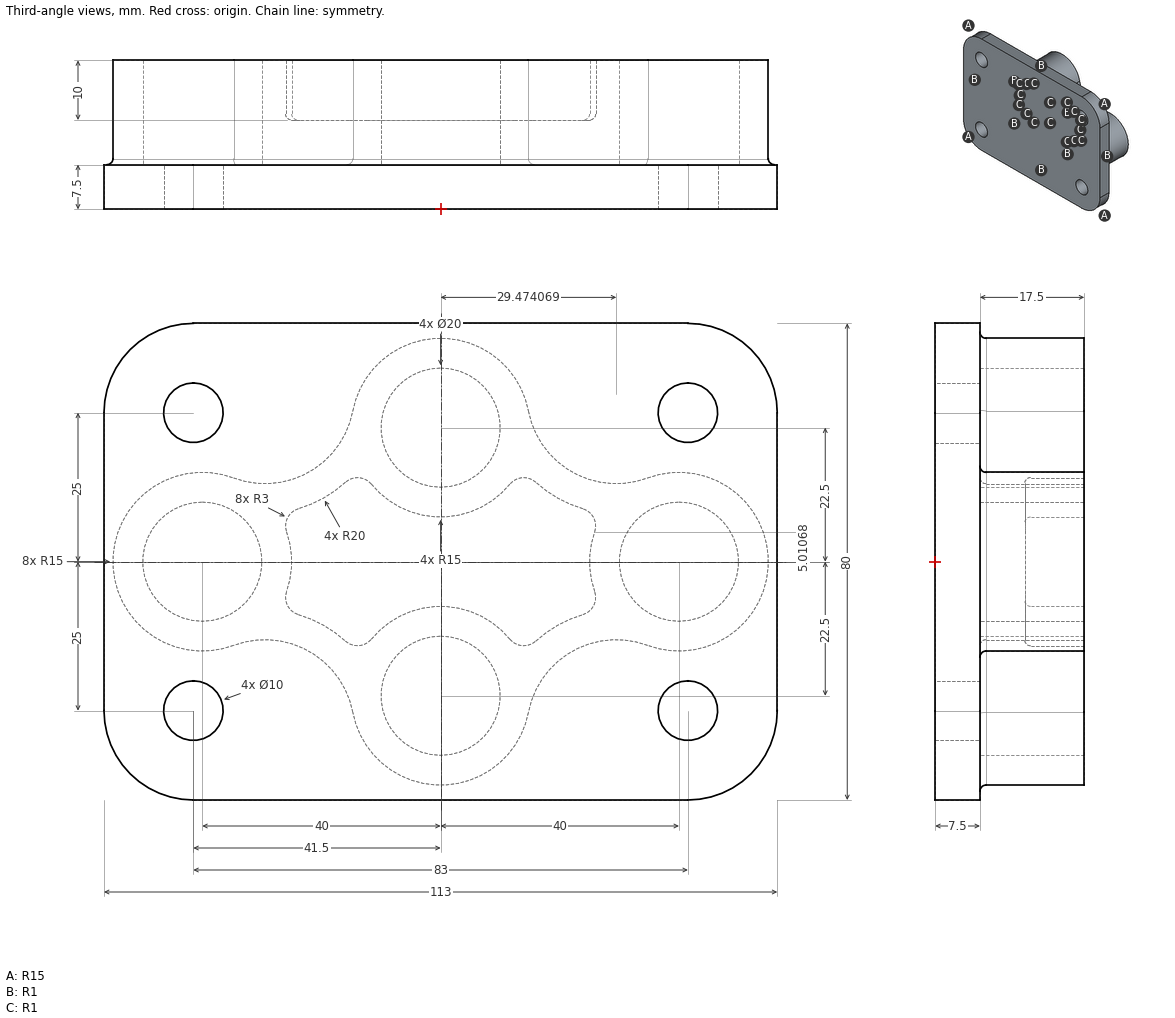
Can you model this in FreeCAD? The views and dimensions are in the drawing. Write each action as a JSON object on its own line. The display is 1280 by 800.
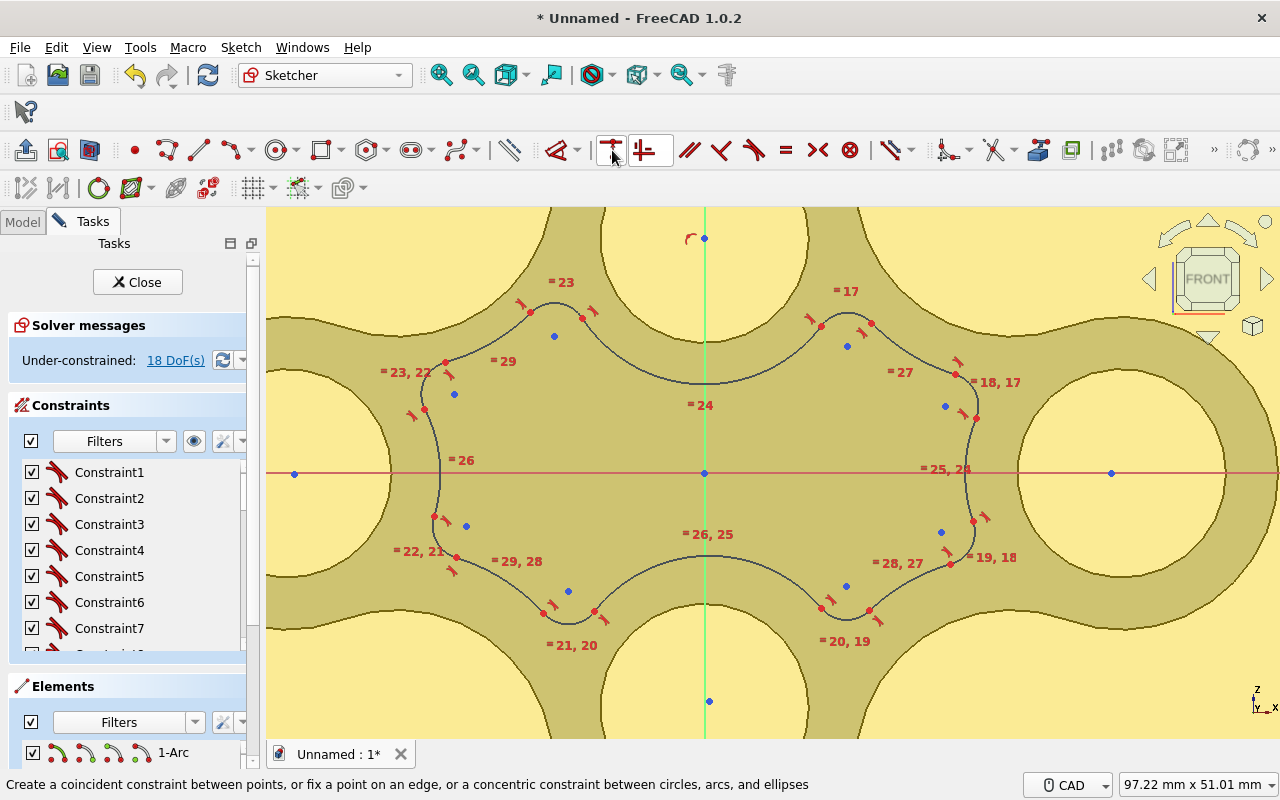
{"action": "left_click", "coordinate": [1111, 474]}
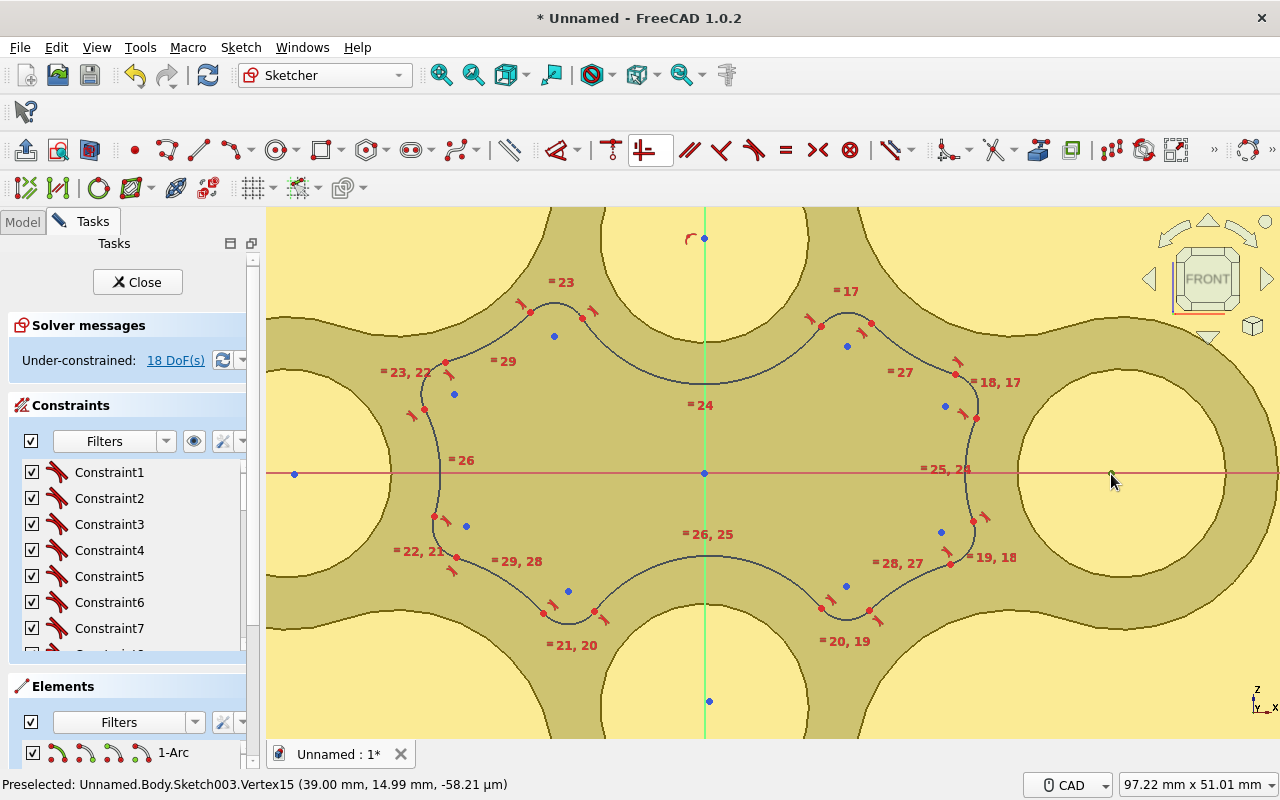
{"action": "left_click", "coordinate": [353, 473]}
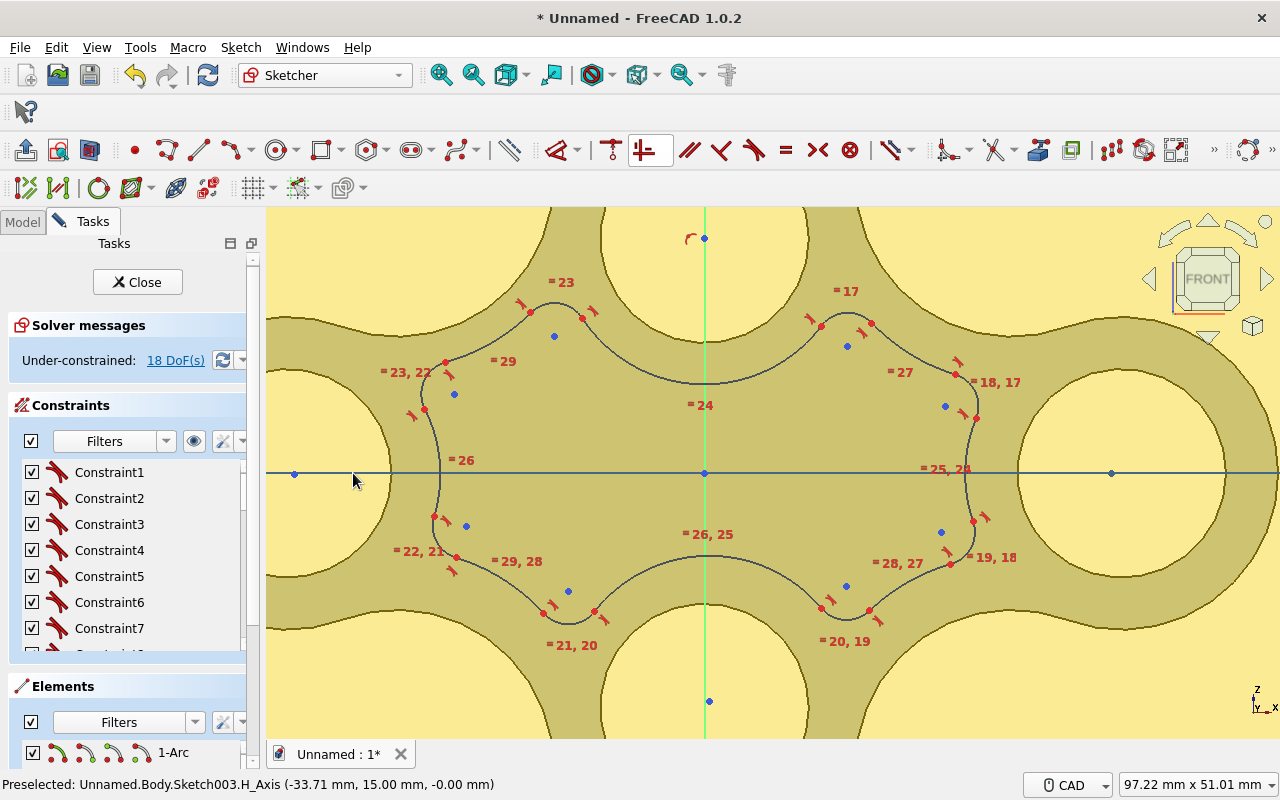
{"action": "key", "text": "c"}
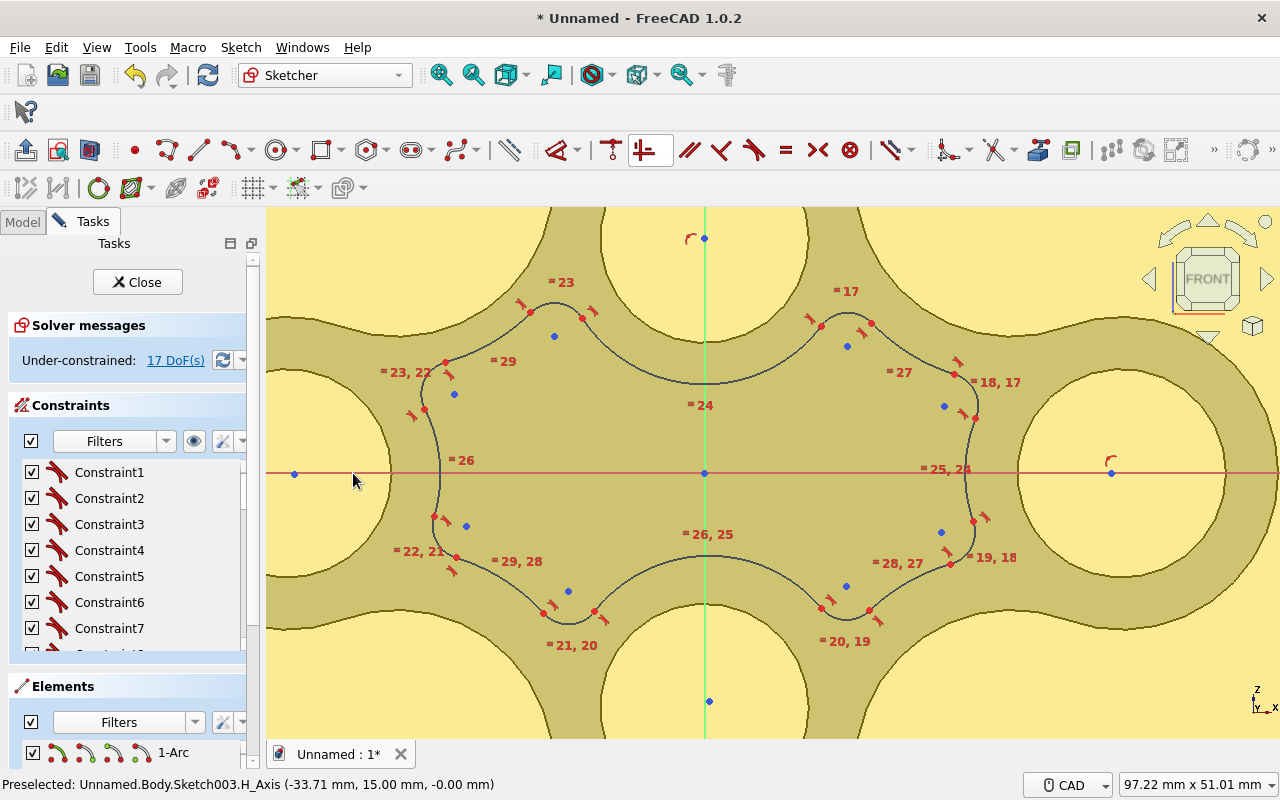
{"action": "left_click", "coordinate": [709, 702]}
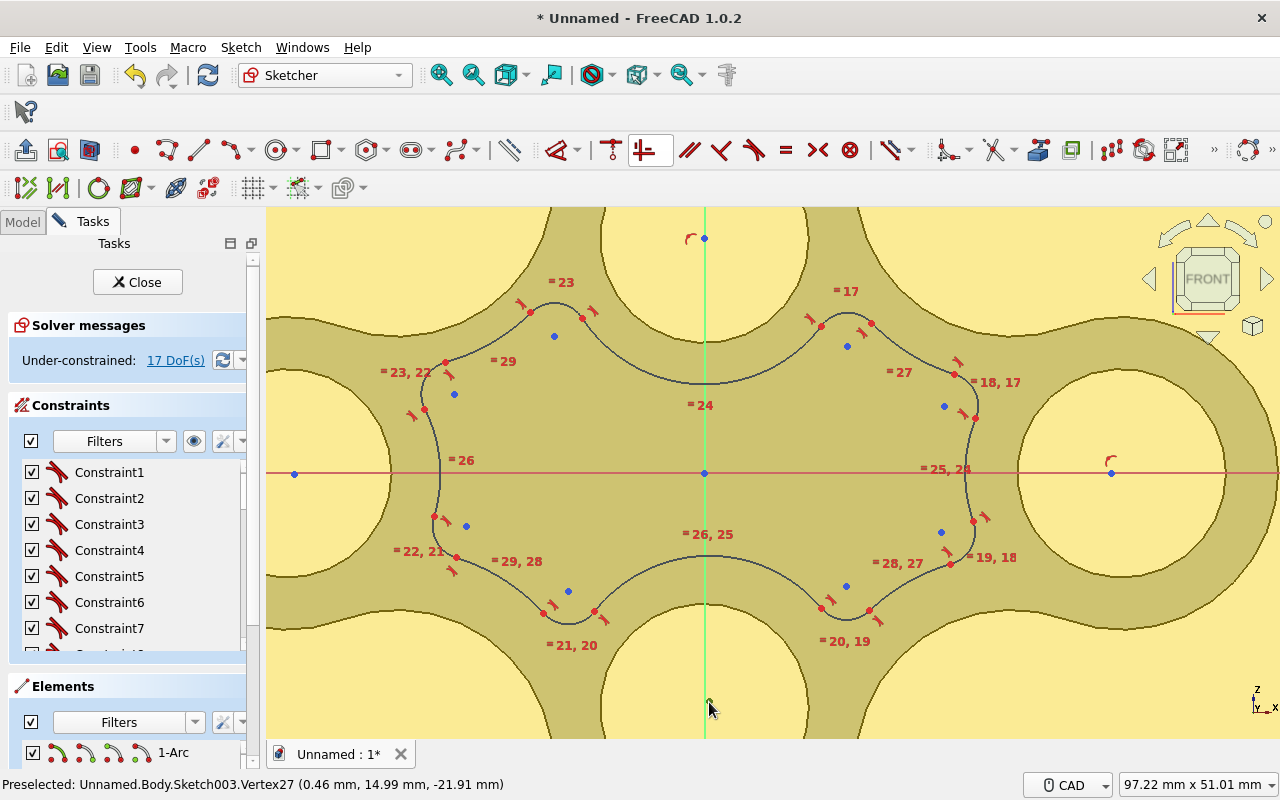
{"action": "left_click", "coordinate": [705, 677]}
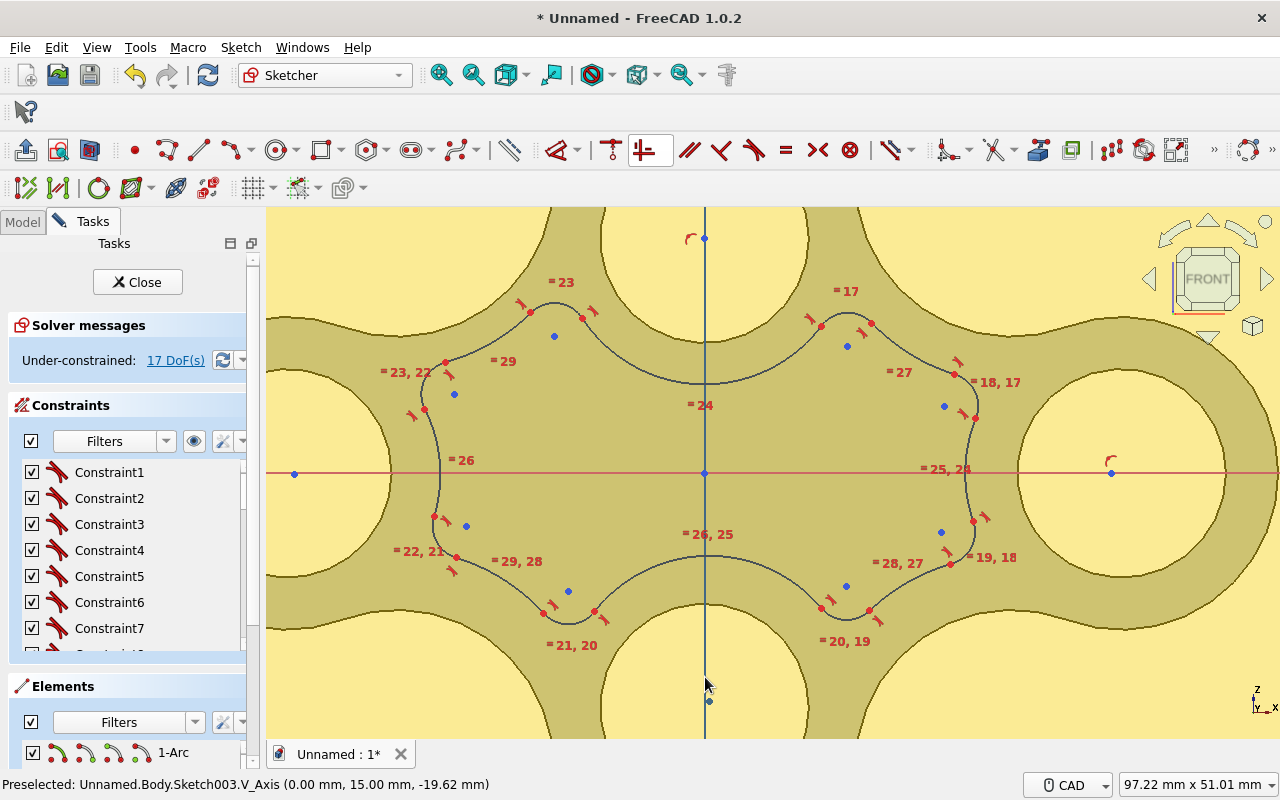
{"action": "left_click", "coordinate": [612, 150]}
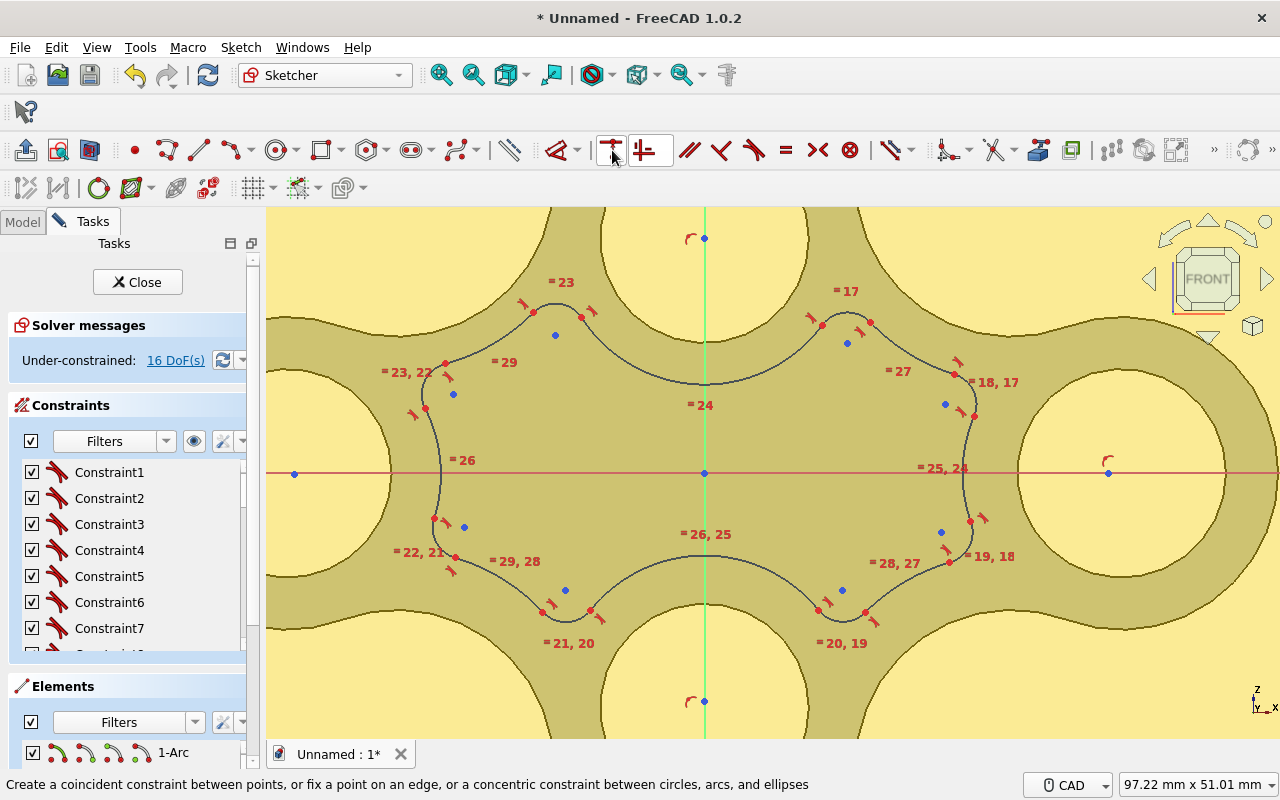
{"action": "left_click", "coordinate": [295, 474]}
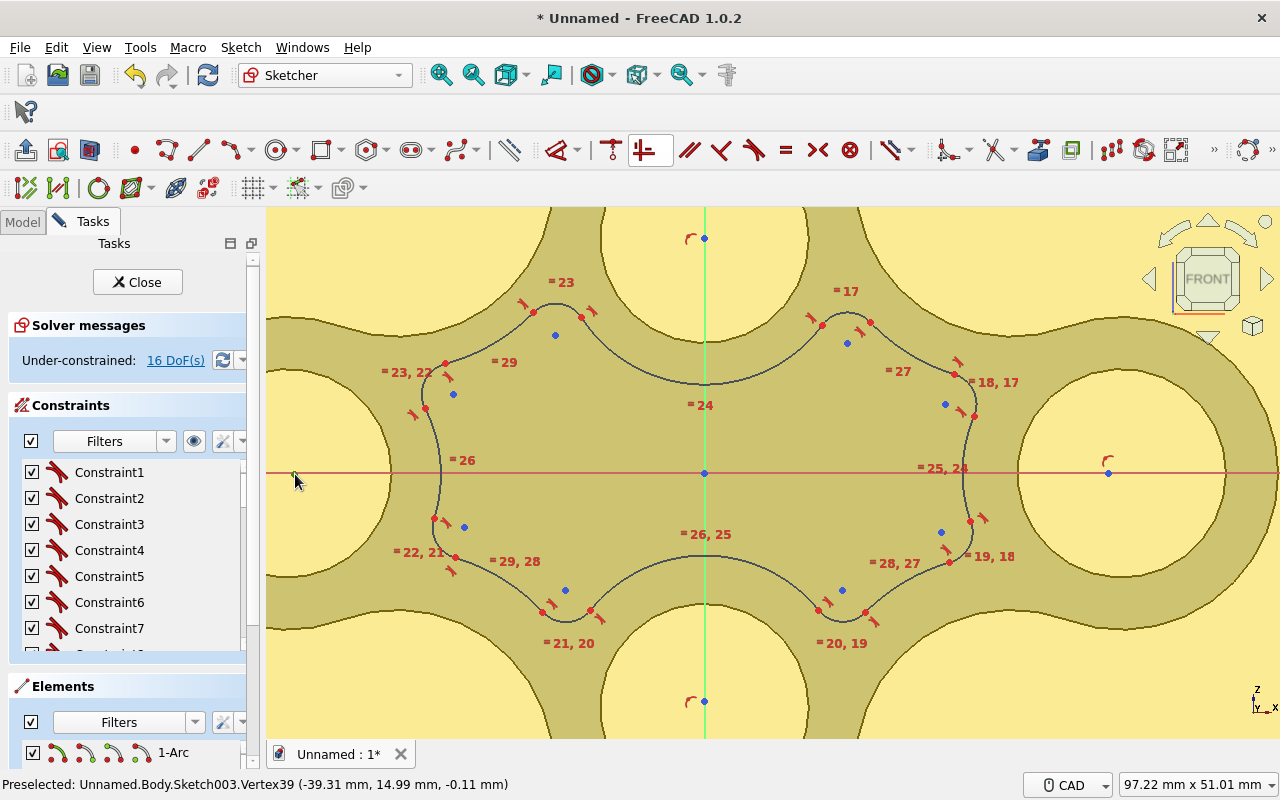
{"action": "left_click", "coordinate": [353, 473]}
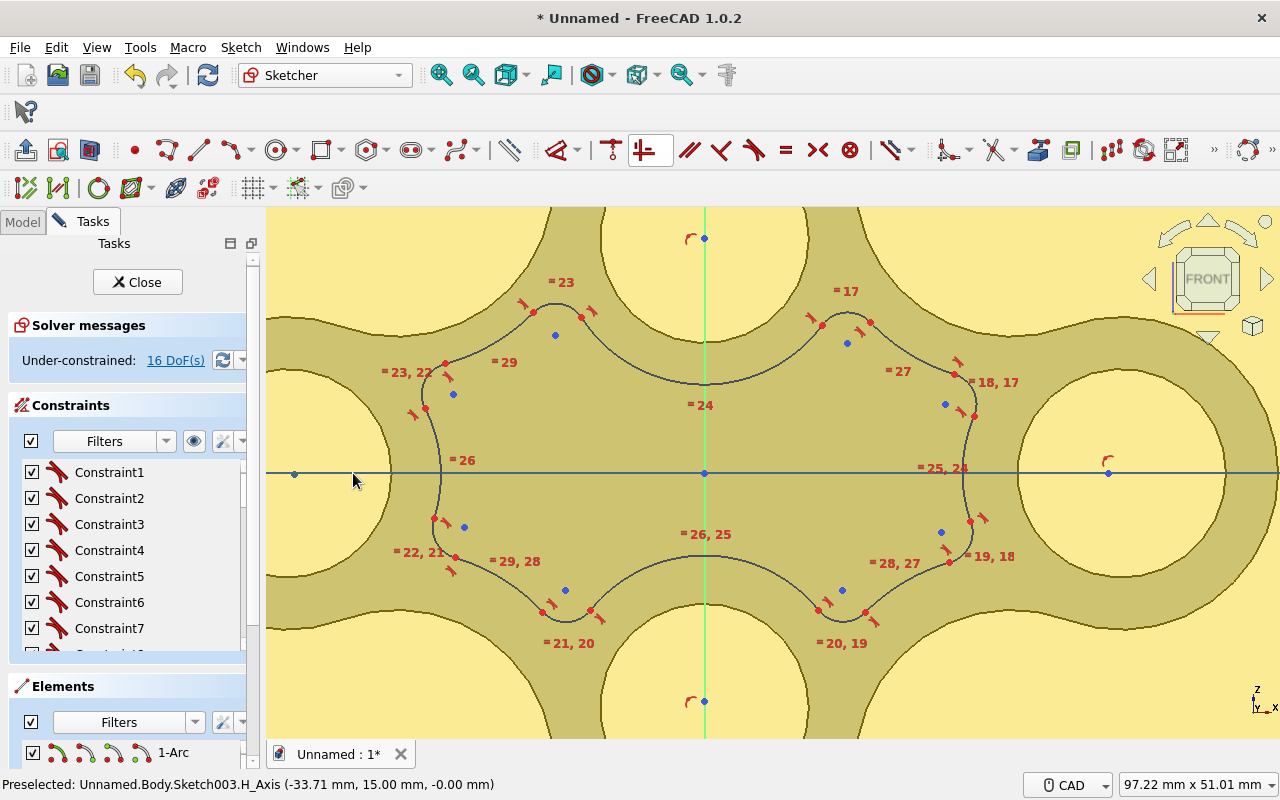
{"action": "left_click", "coordinate": [612, 150]}